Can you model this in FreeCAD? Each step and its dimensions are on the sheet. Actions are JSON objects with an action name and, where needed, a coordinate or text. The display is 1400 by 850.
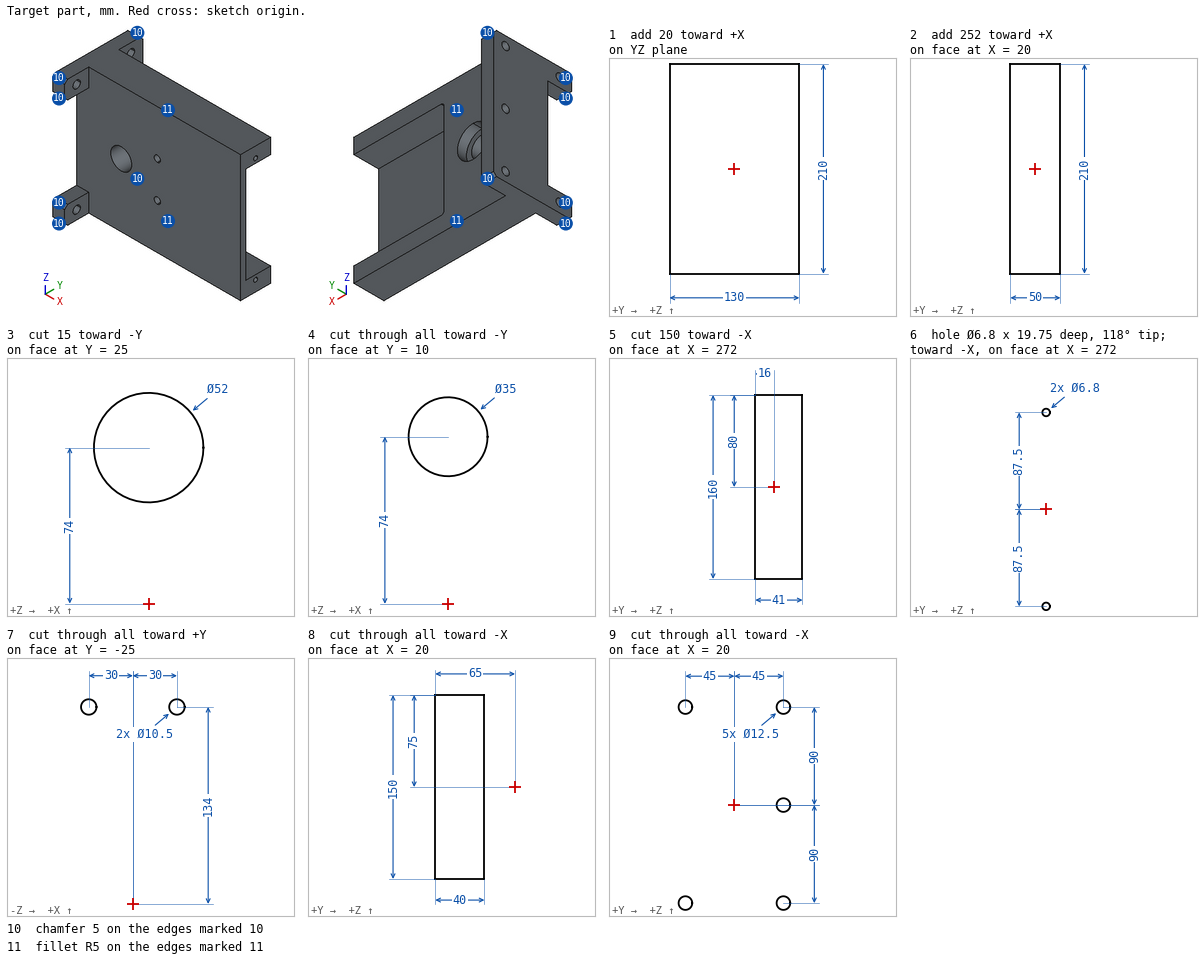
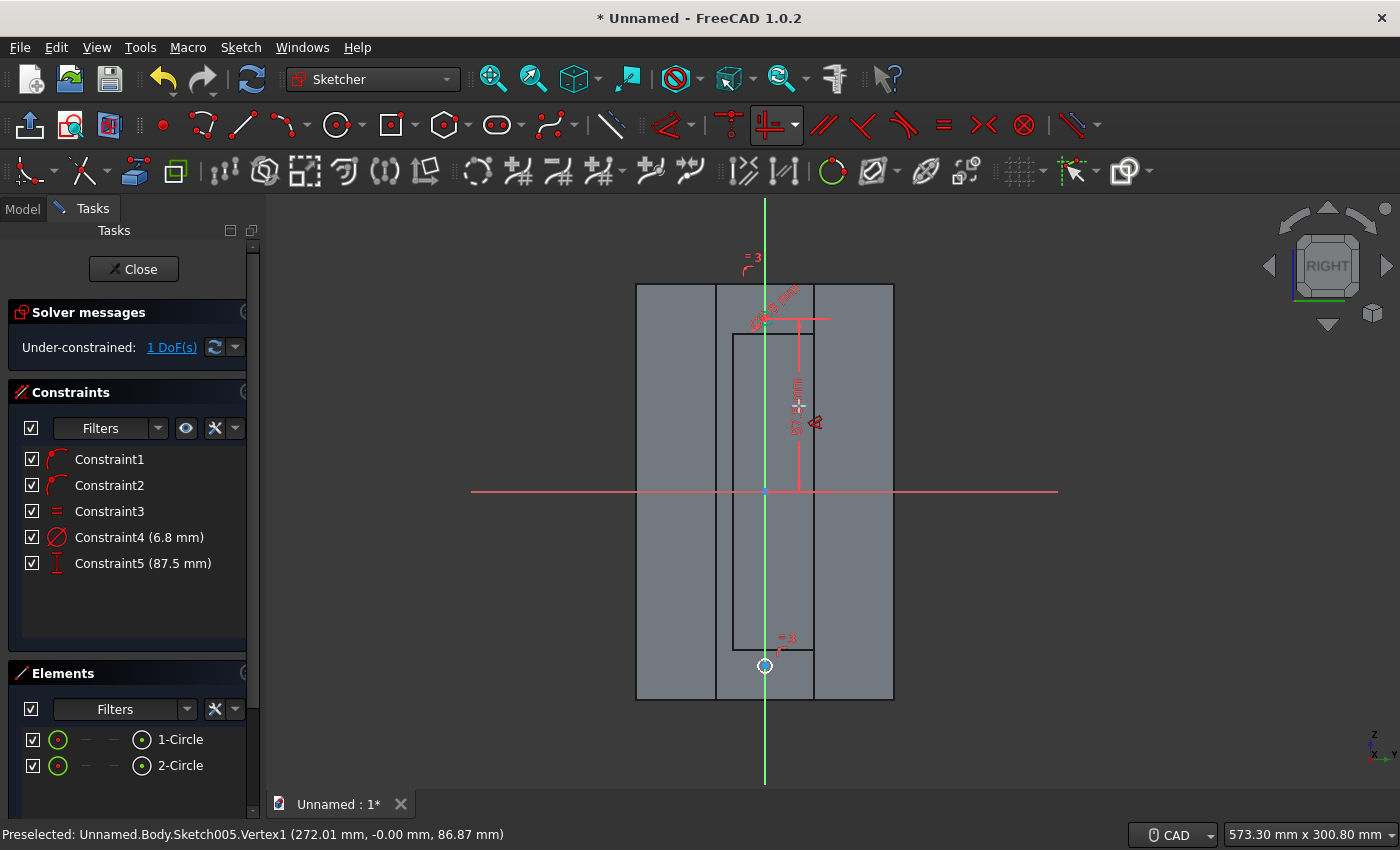
{"action": "left_click", "coordinate": [765, 666]}
{"action": "left_click", "coordinate": [799, 579]}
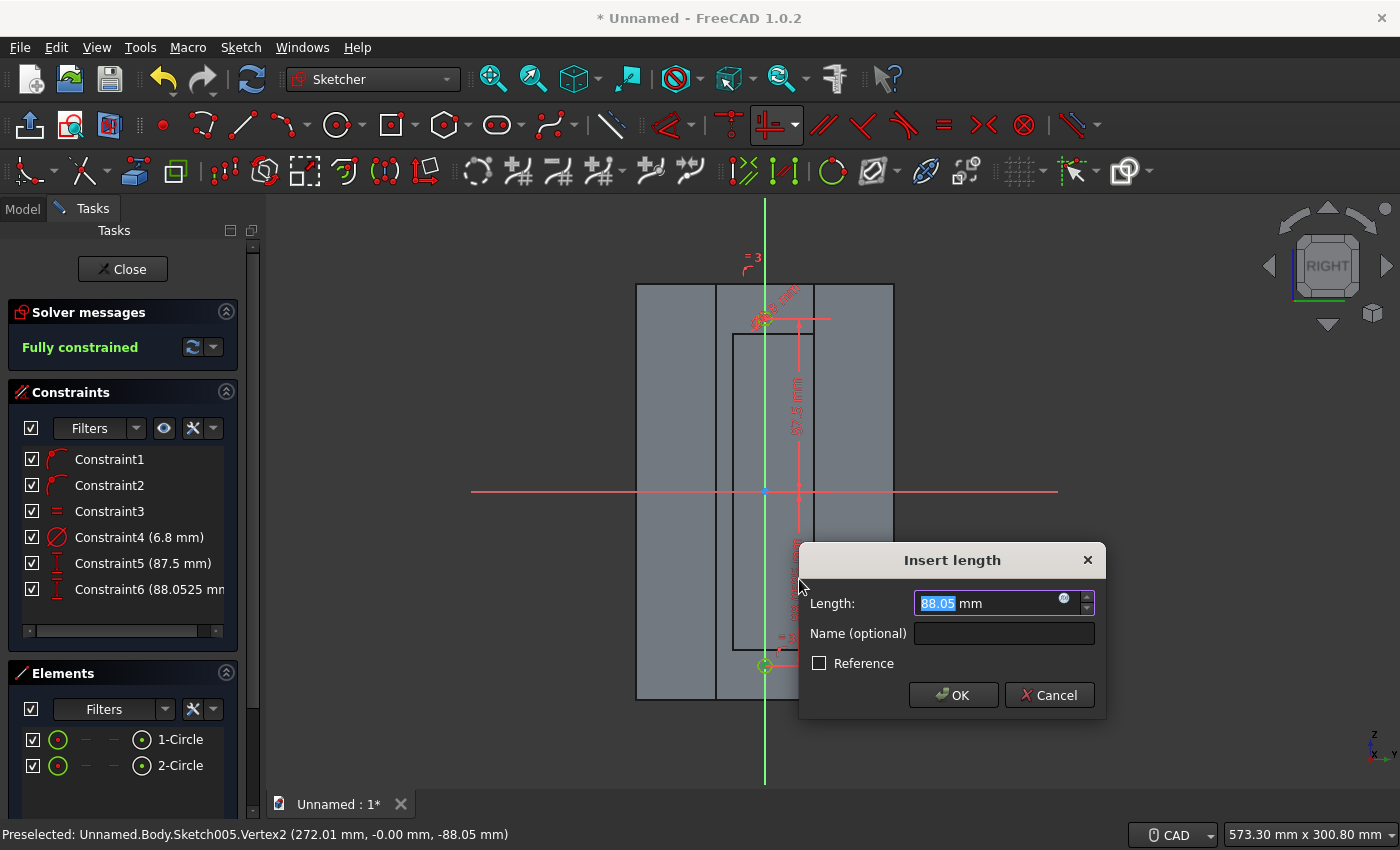
{"action": "type", "text": "87.5"}
{"action": "key", "text": "Return"}
{"action": "key", "text": "Escape"}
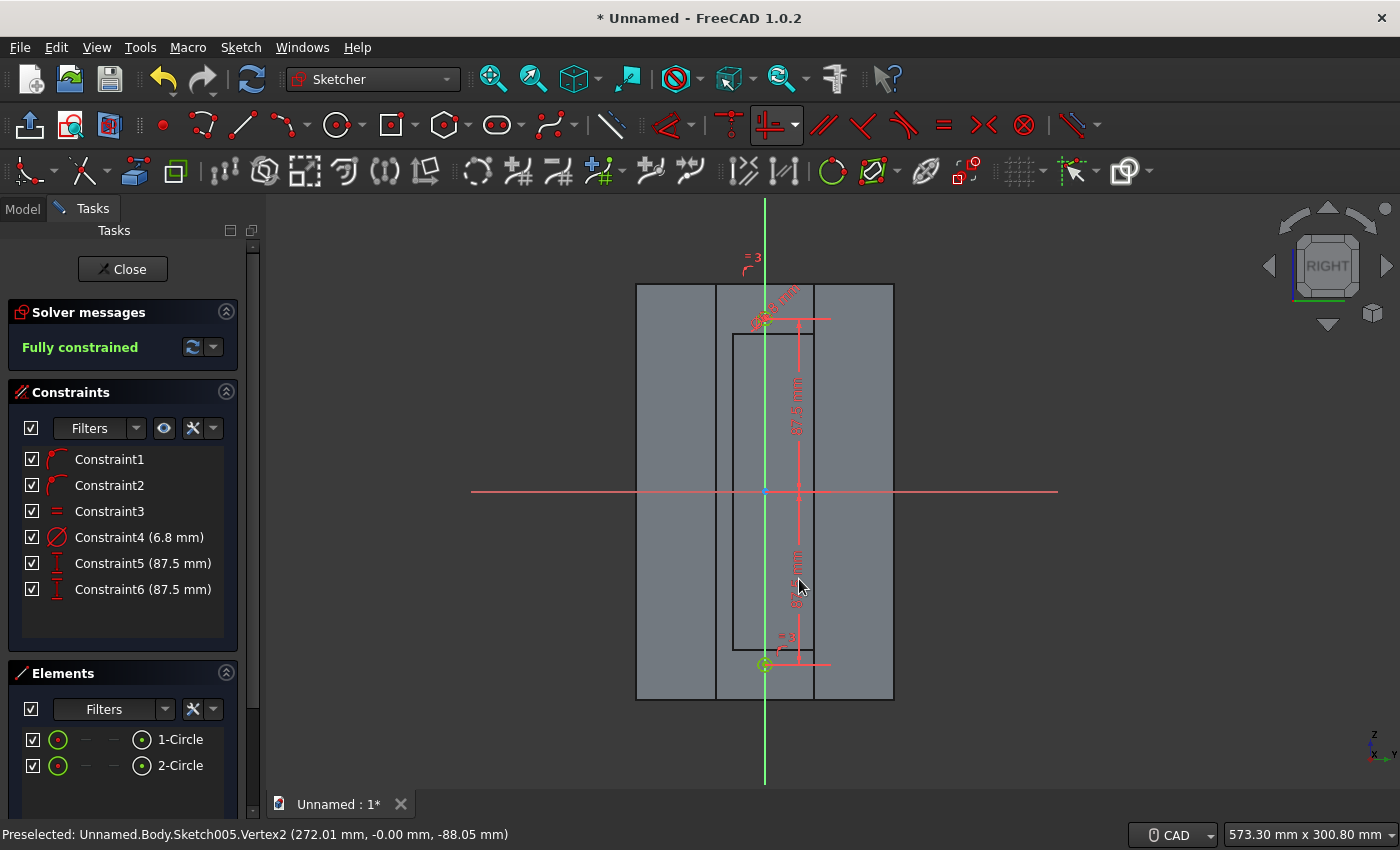
{"action": "left_click", "coordinate": [123, 269]}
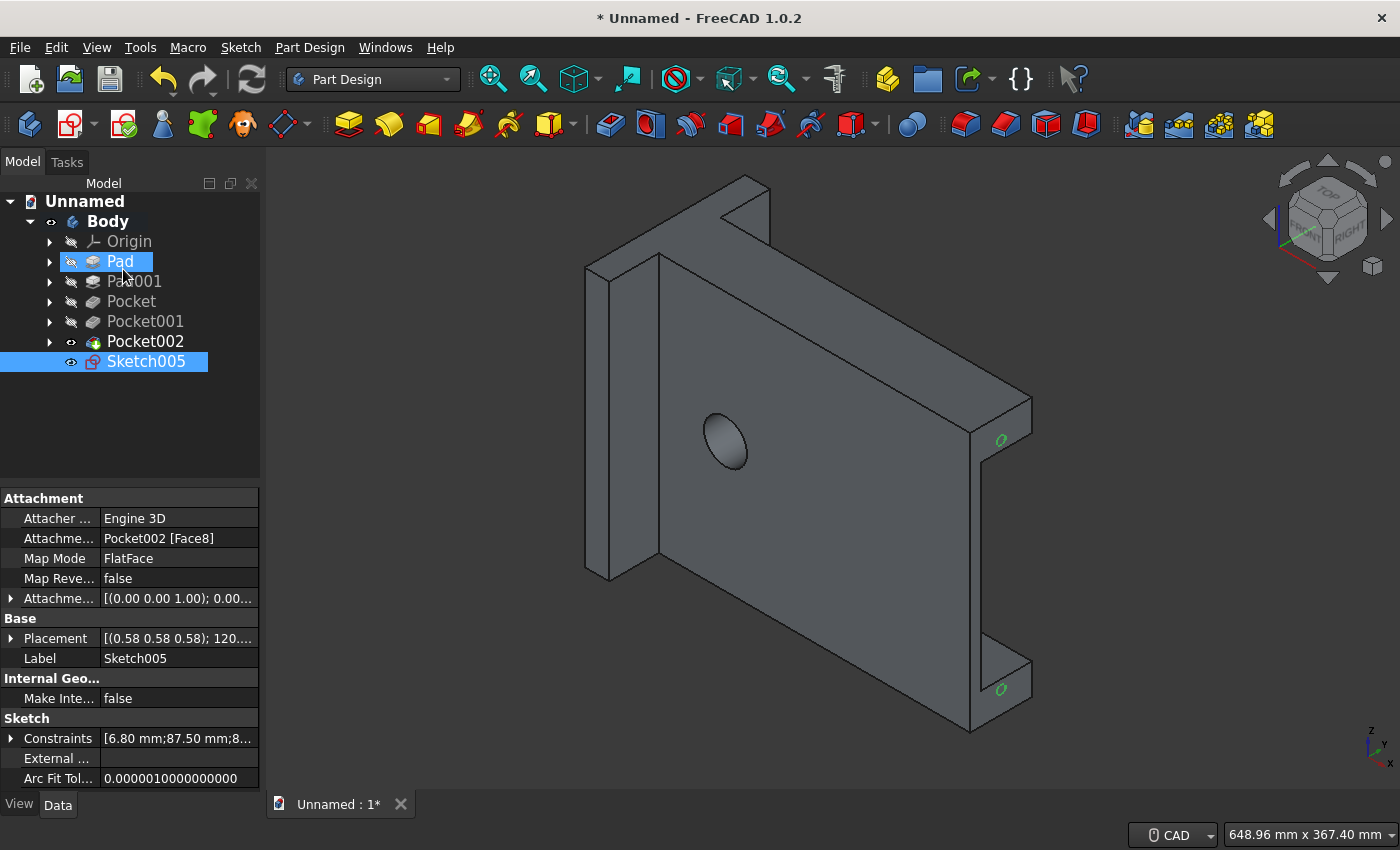
{"action": "left_click", "coordinate": [652, 124]}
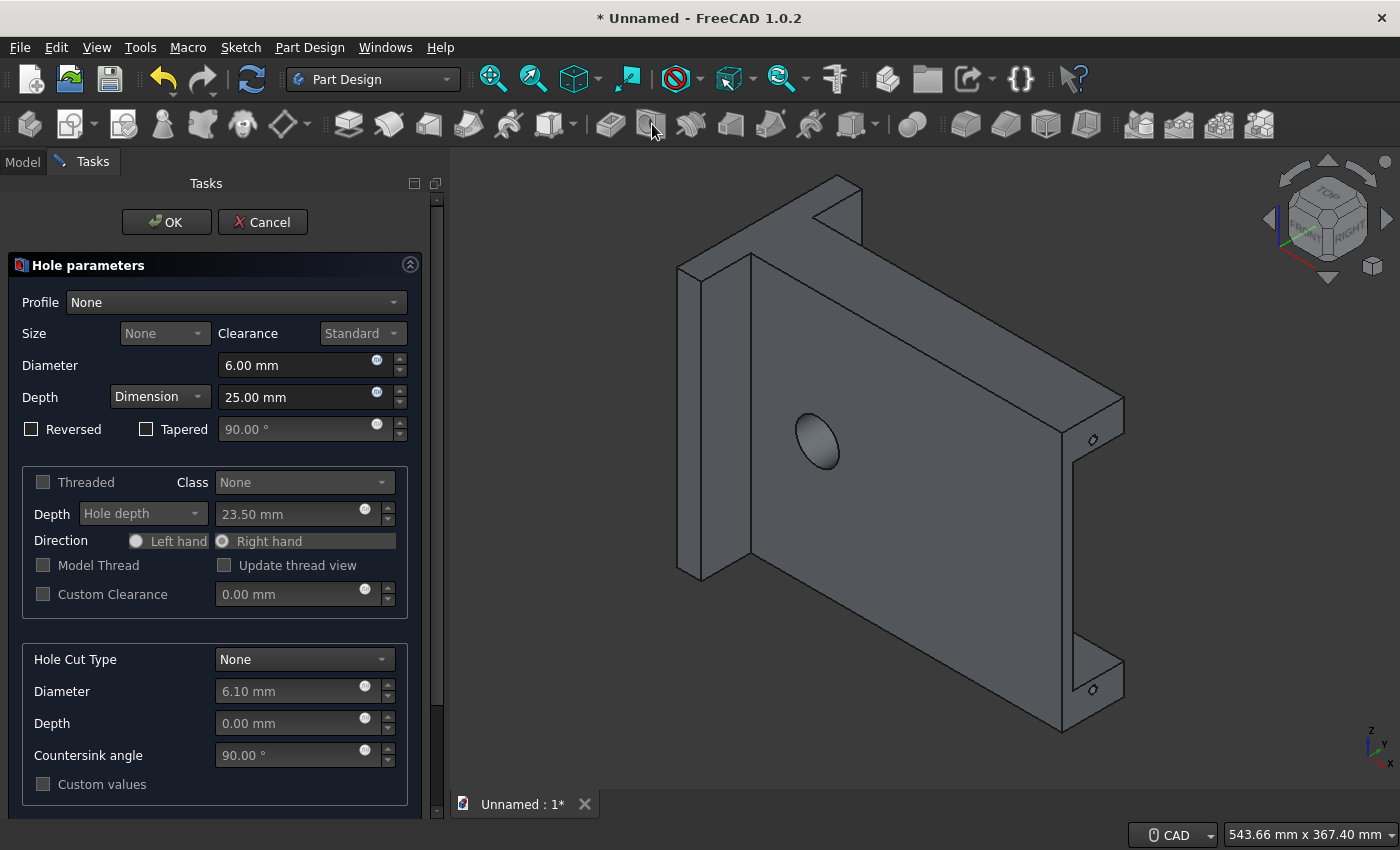
{"action": "triple_click", "coordinate": [305, 365]}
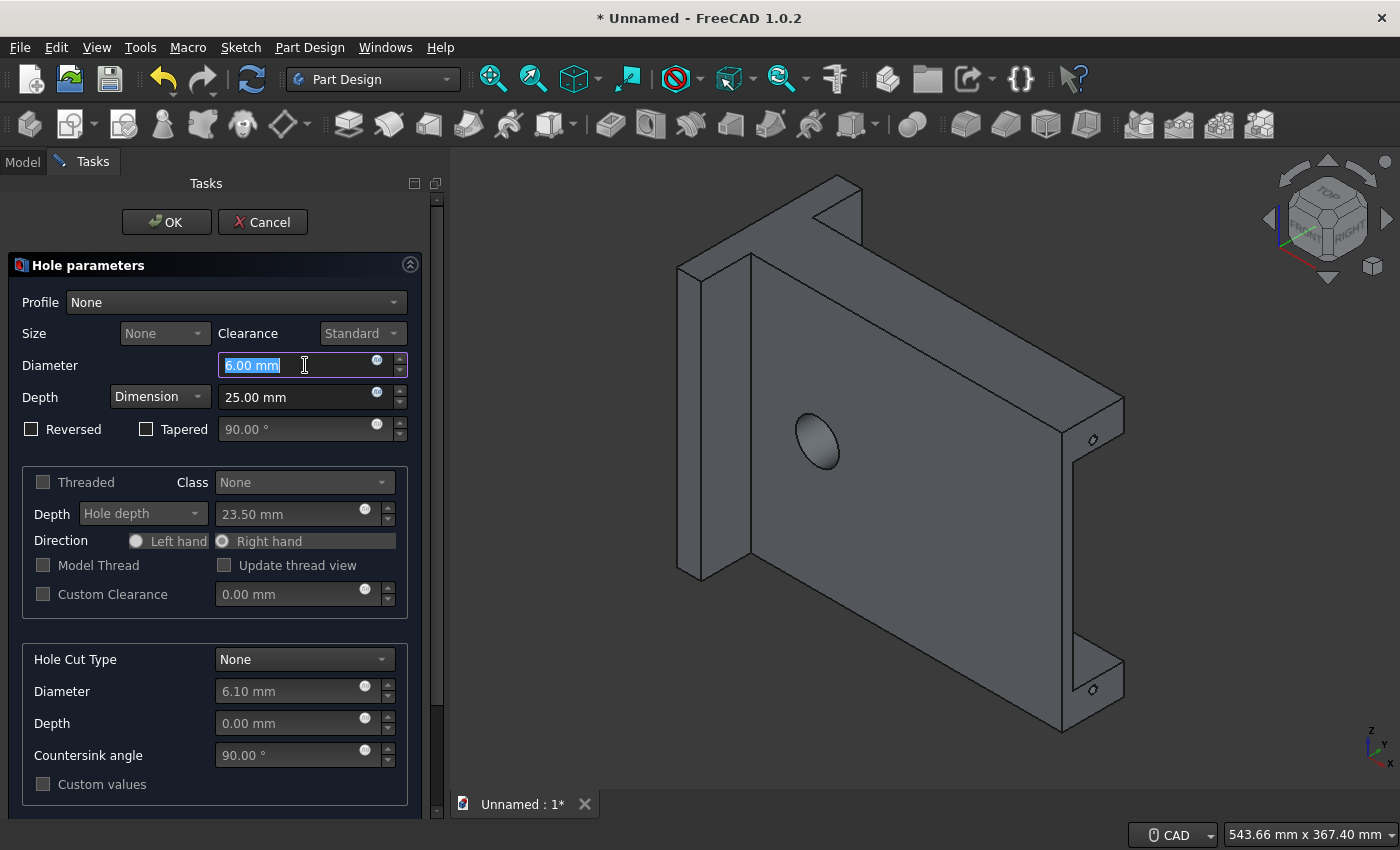
{"action": "type", "text": "6.8"}
{"action": "key", "text": "Tab"}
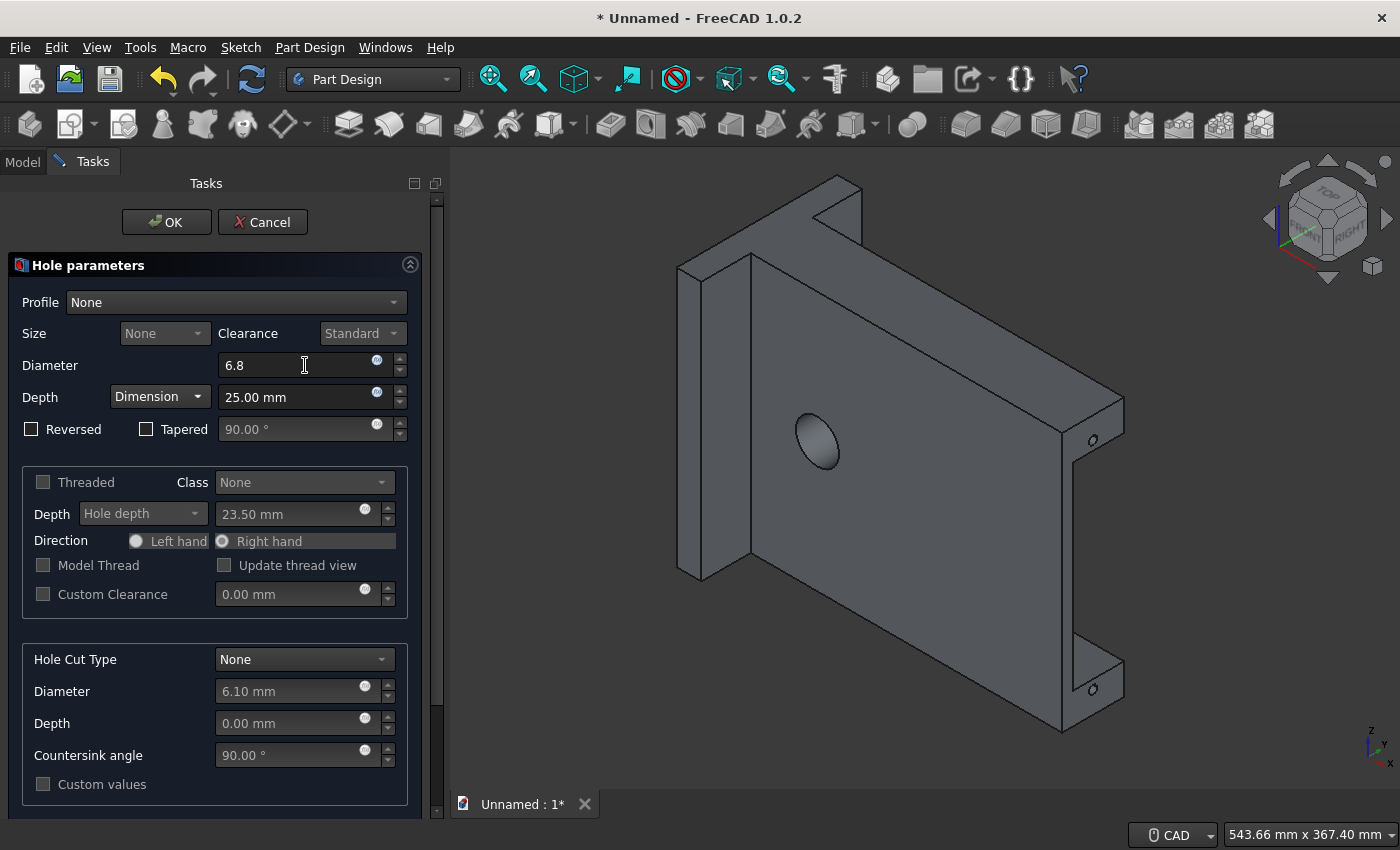
{"action": "triple_click", "coordinate": [305, 397]}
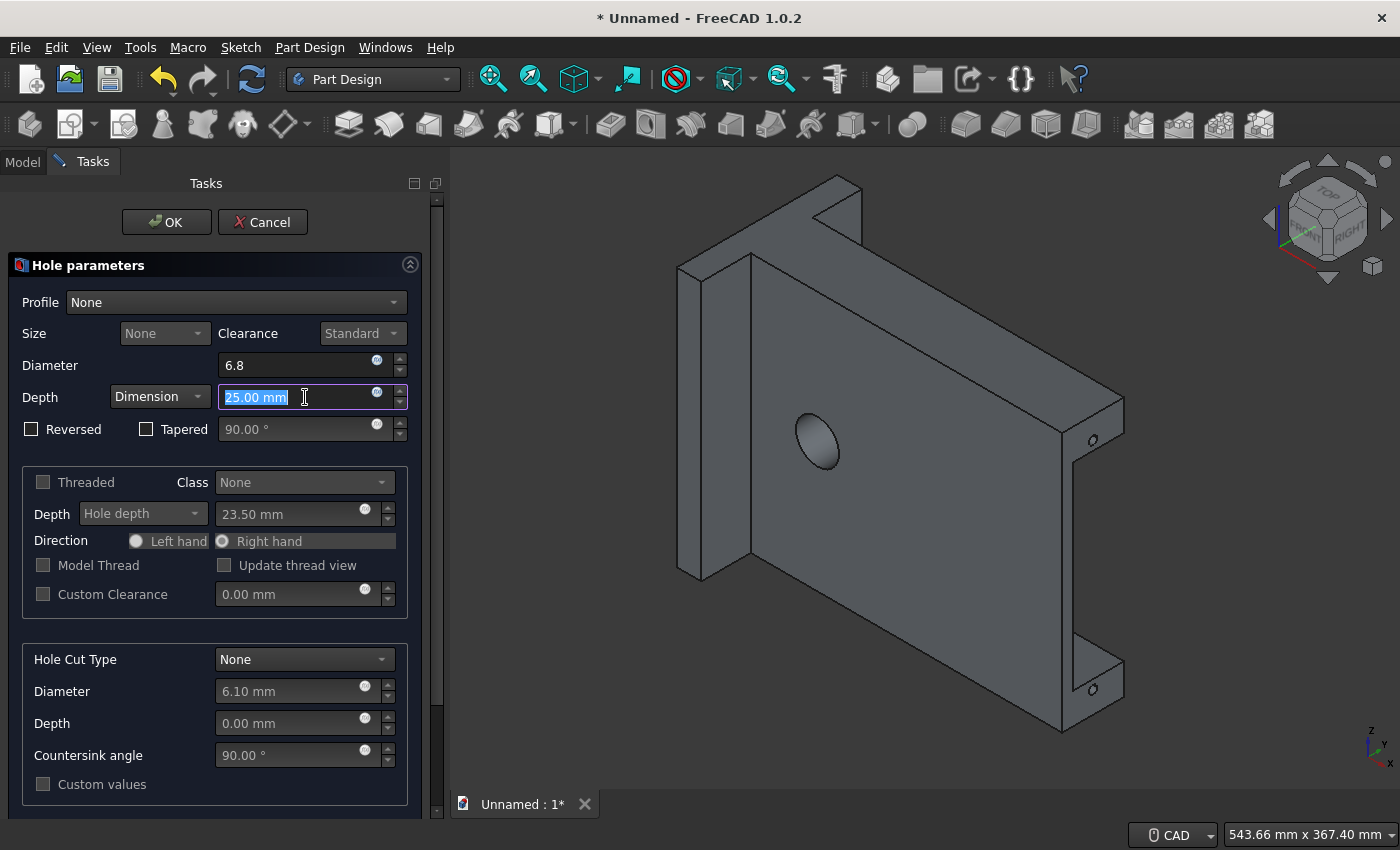
{"action": "type", "text": "19.75"}
{"action": "key", "text": "Tab"}